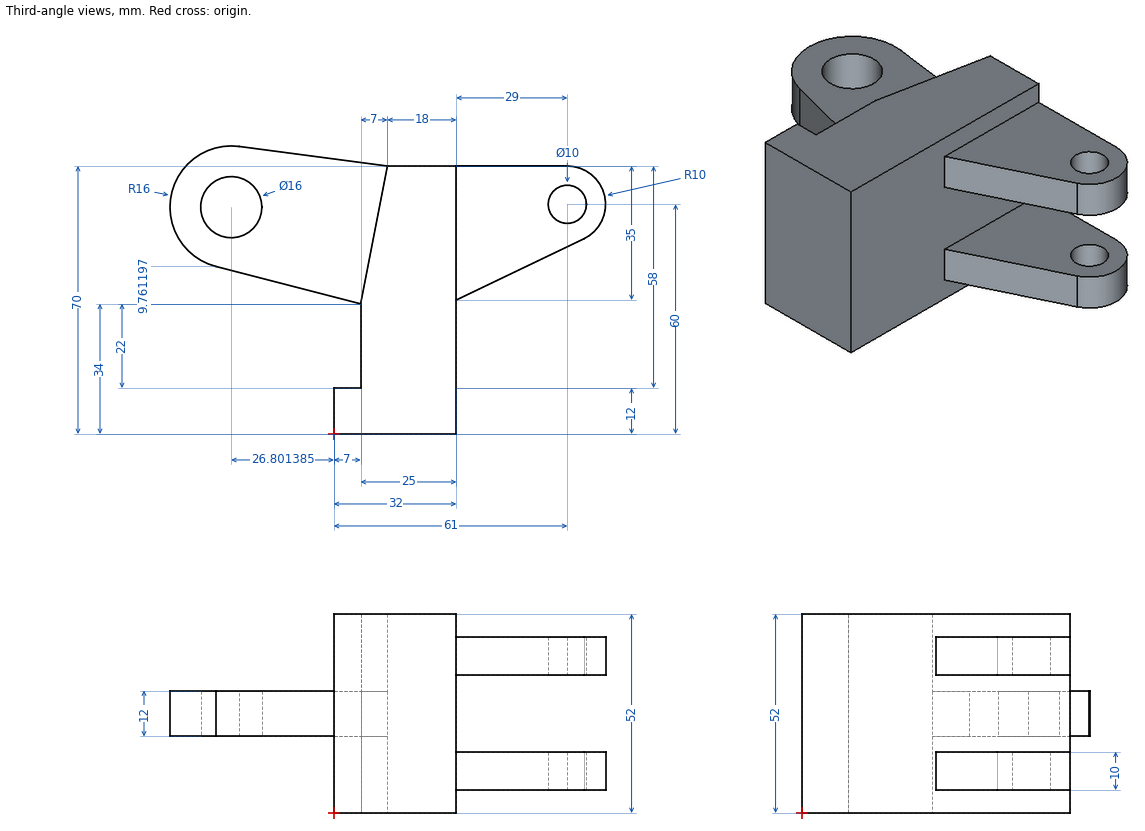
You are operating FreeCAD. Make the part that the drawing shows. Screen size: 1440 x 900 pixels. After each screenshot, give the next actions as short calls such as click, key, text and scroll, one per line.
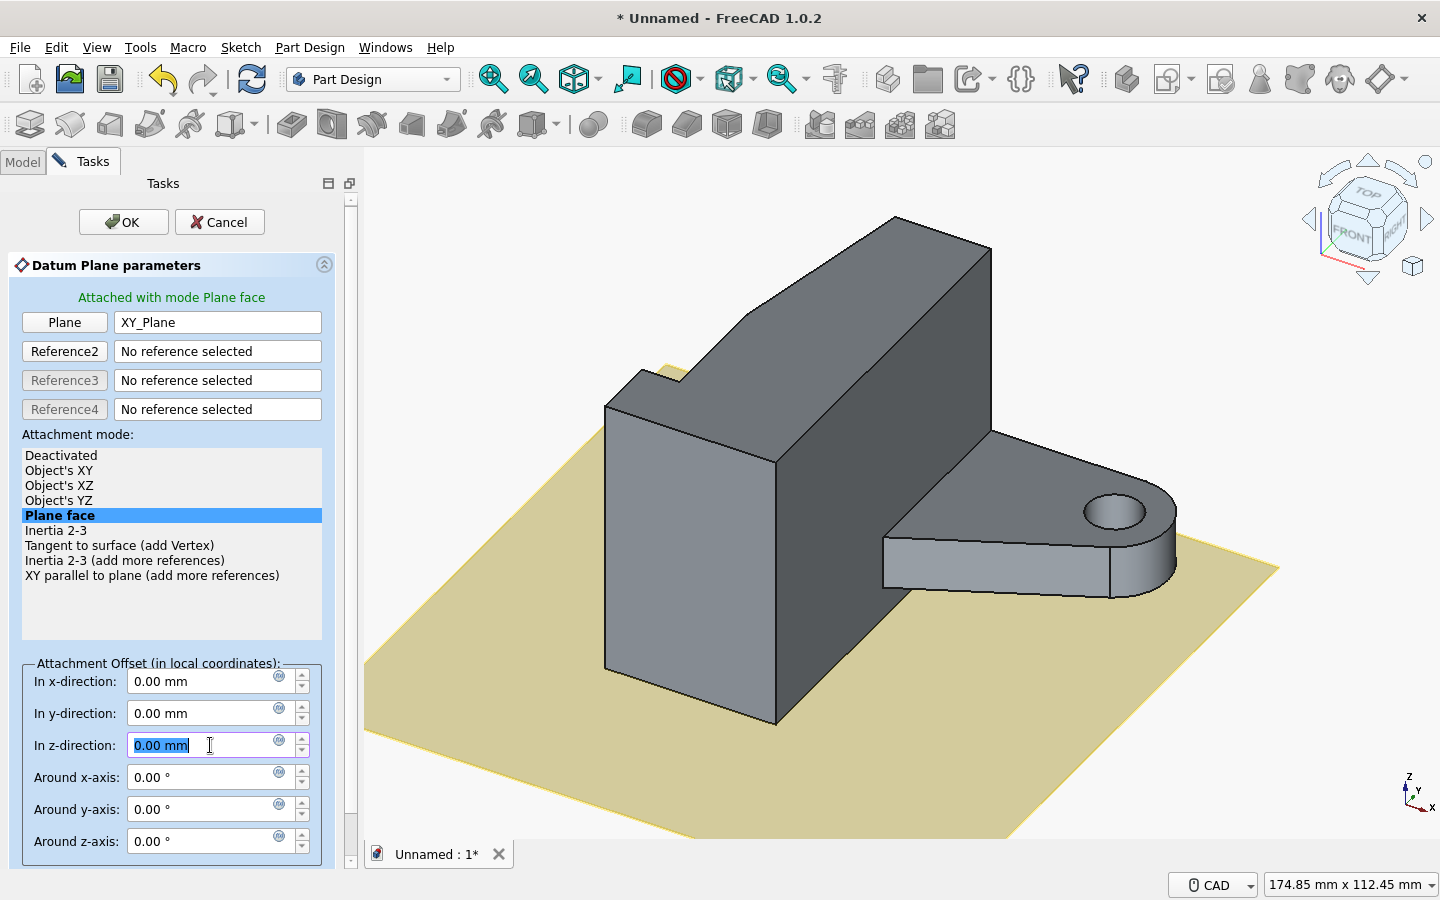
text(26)
key(Tab)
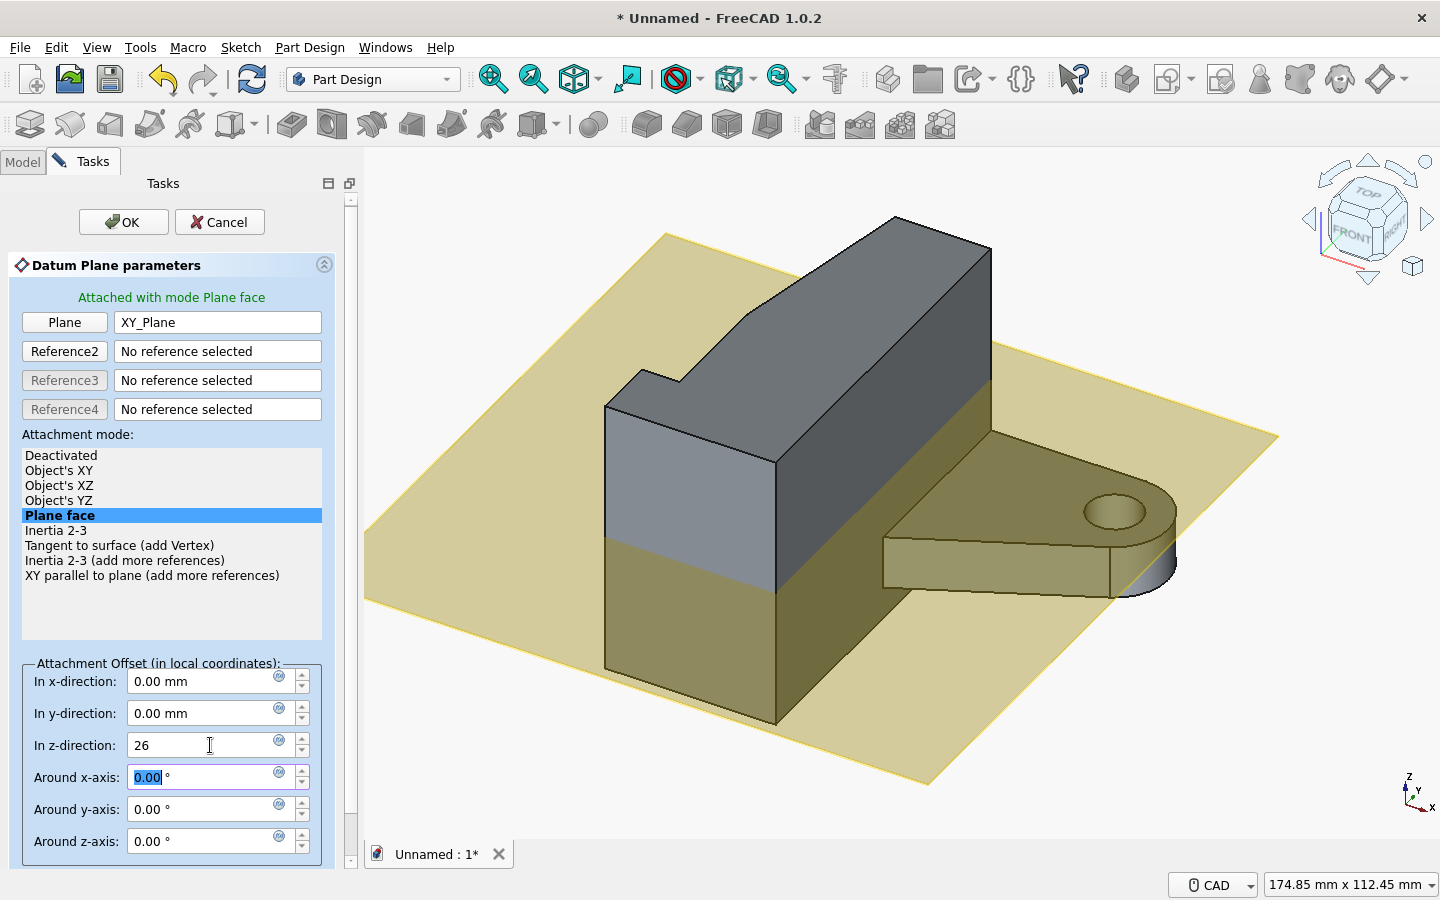
click(124, 222)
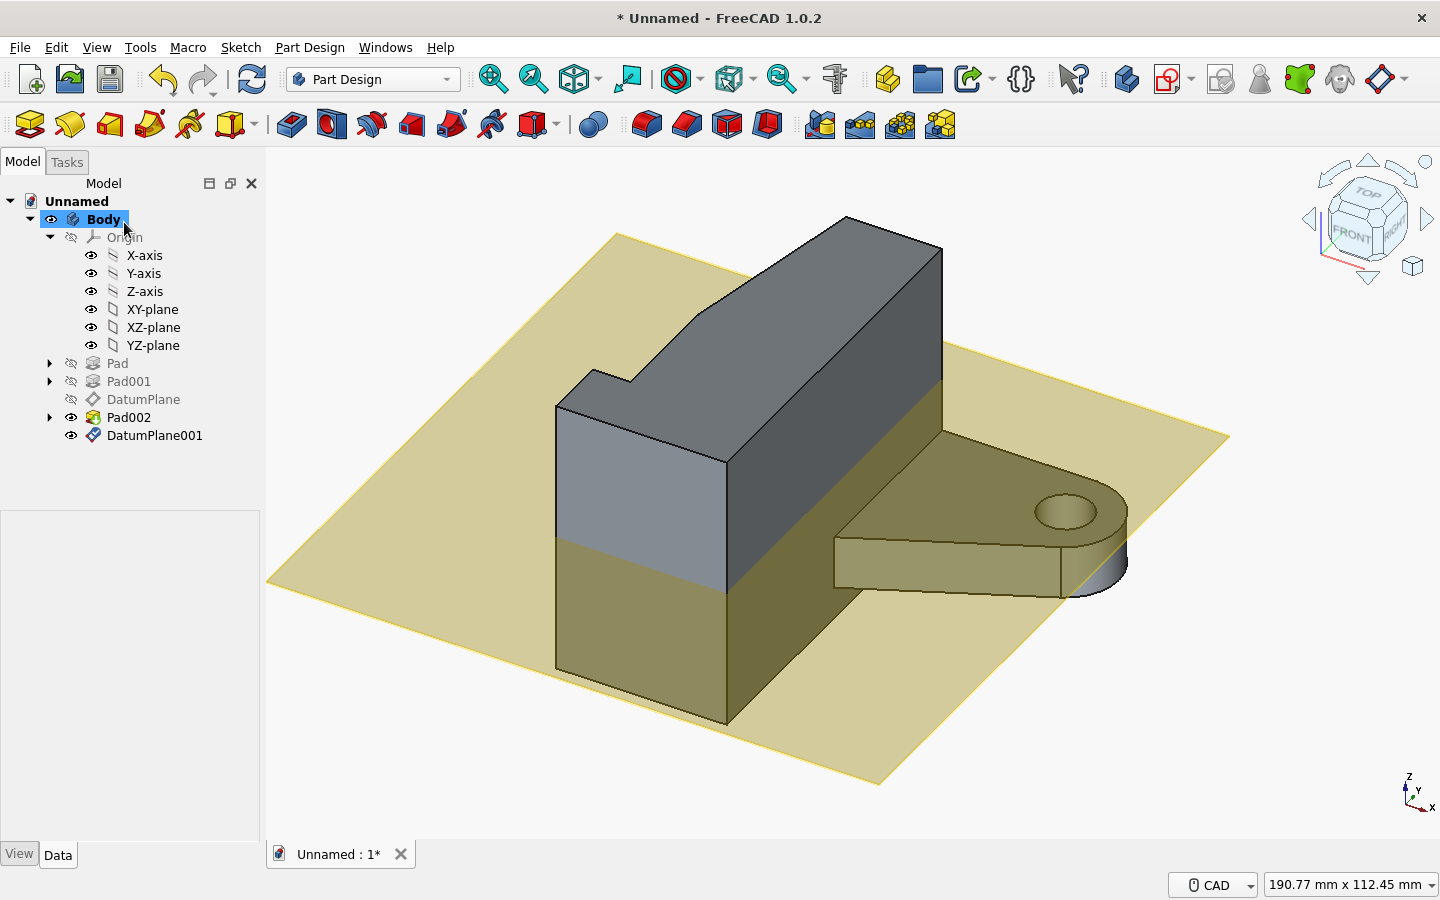
click(116, 417)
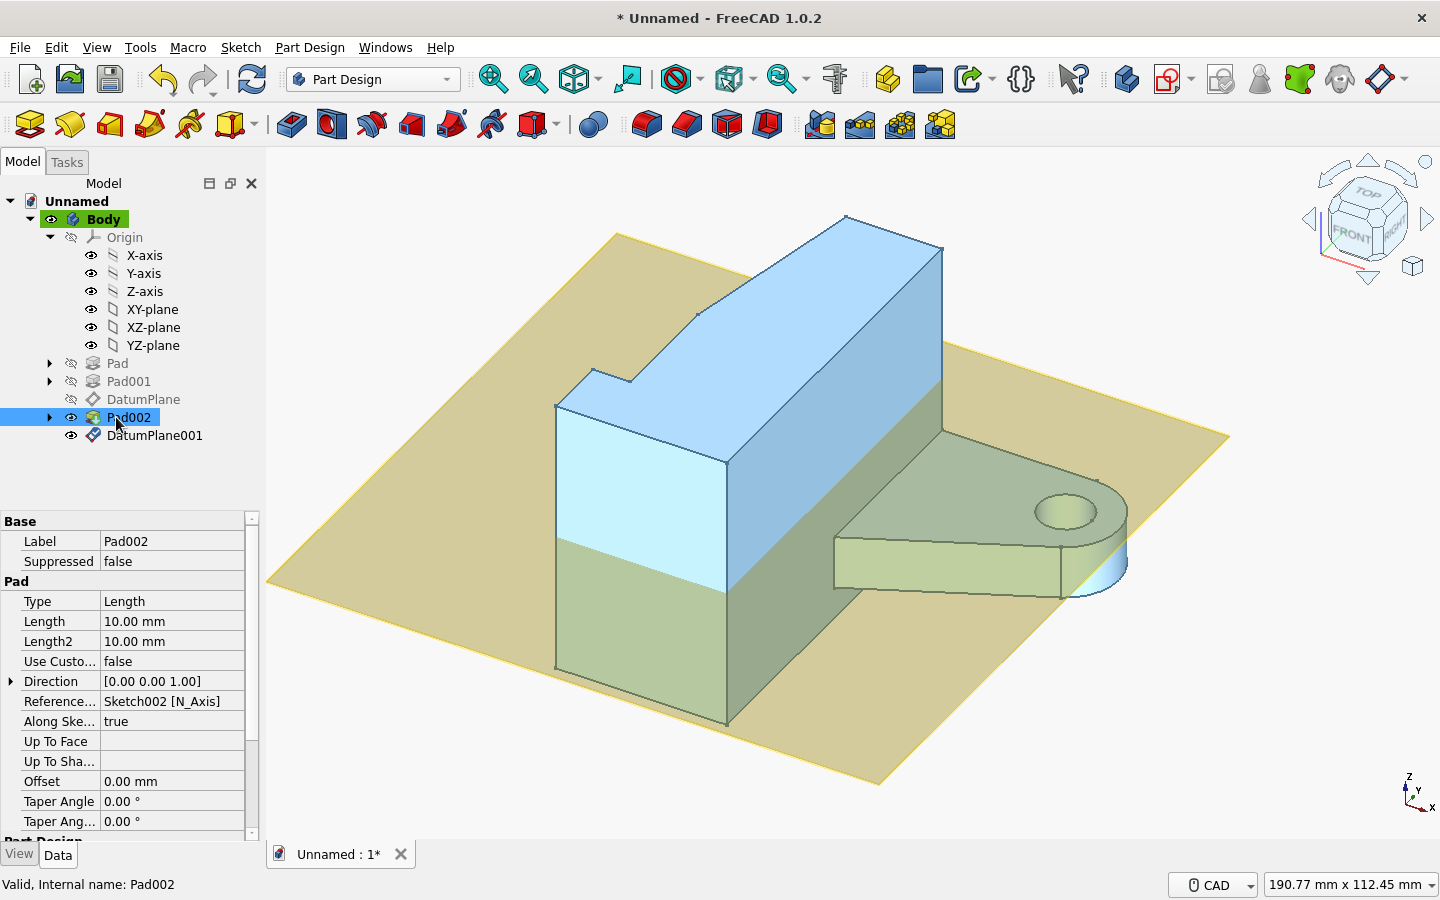
click(820, 124)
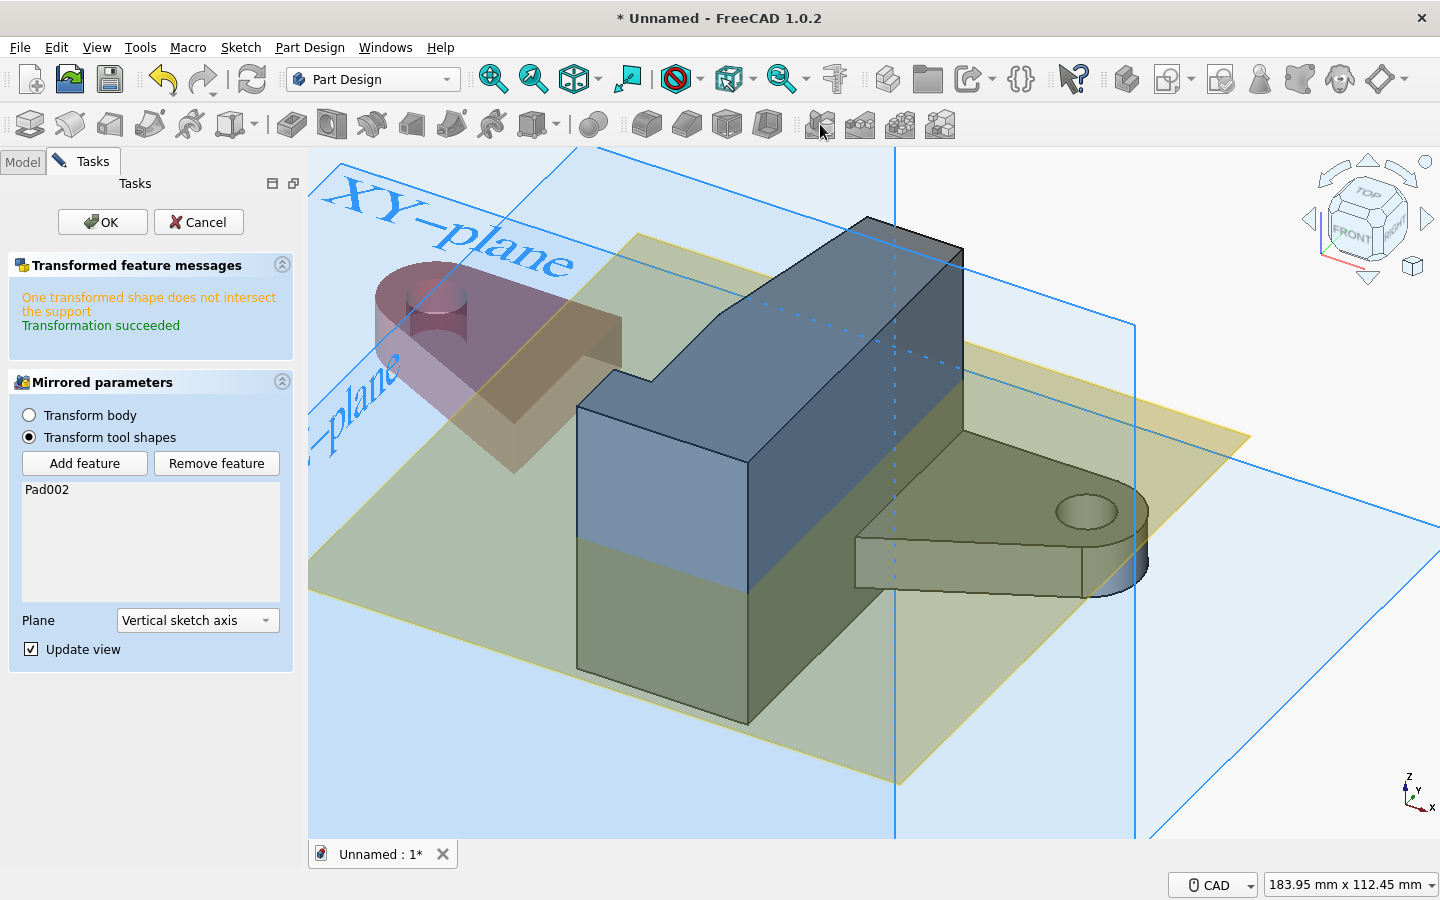
click(198, 620)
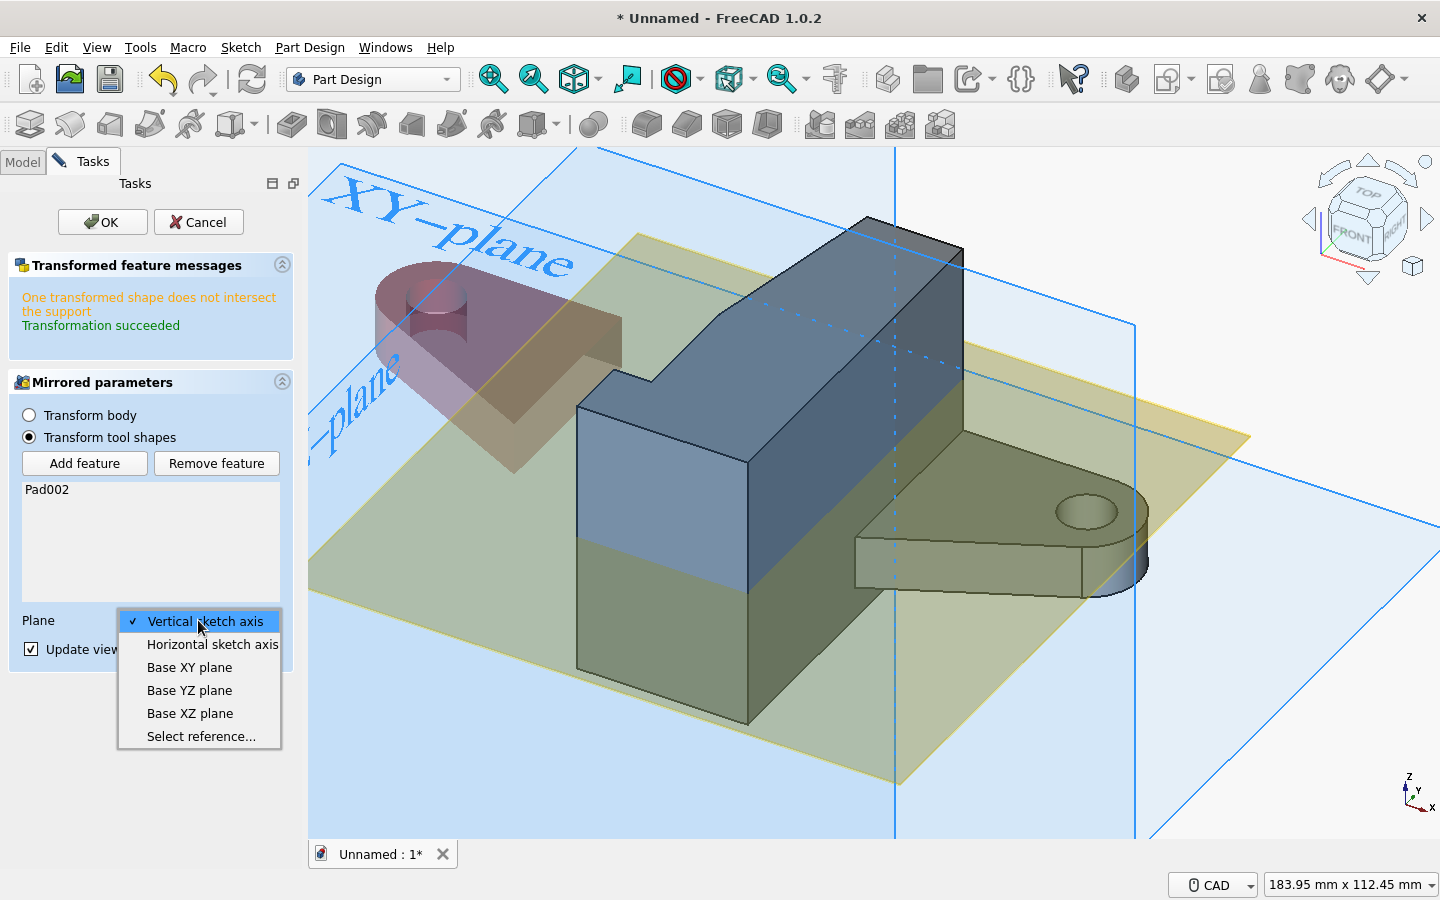
click(198, 736)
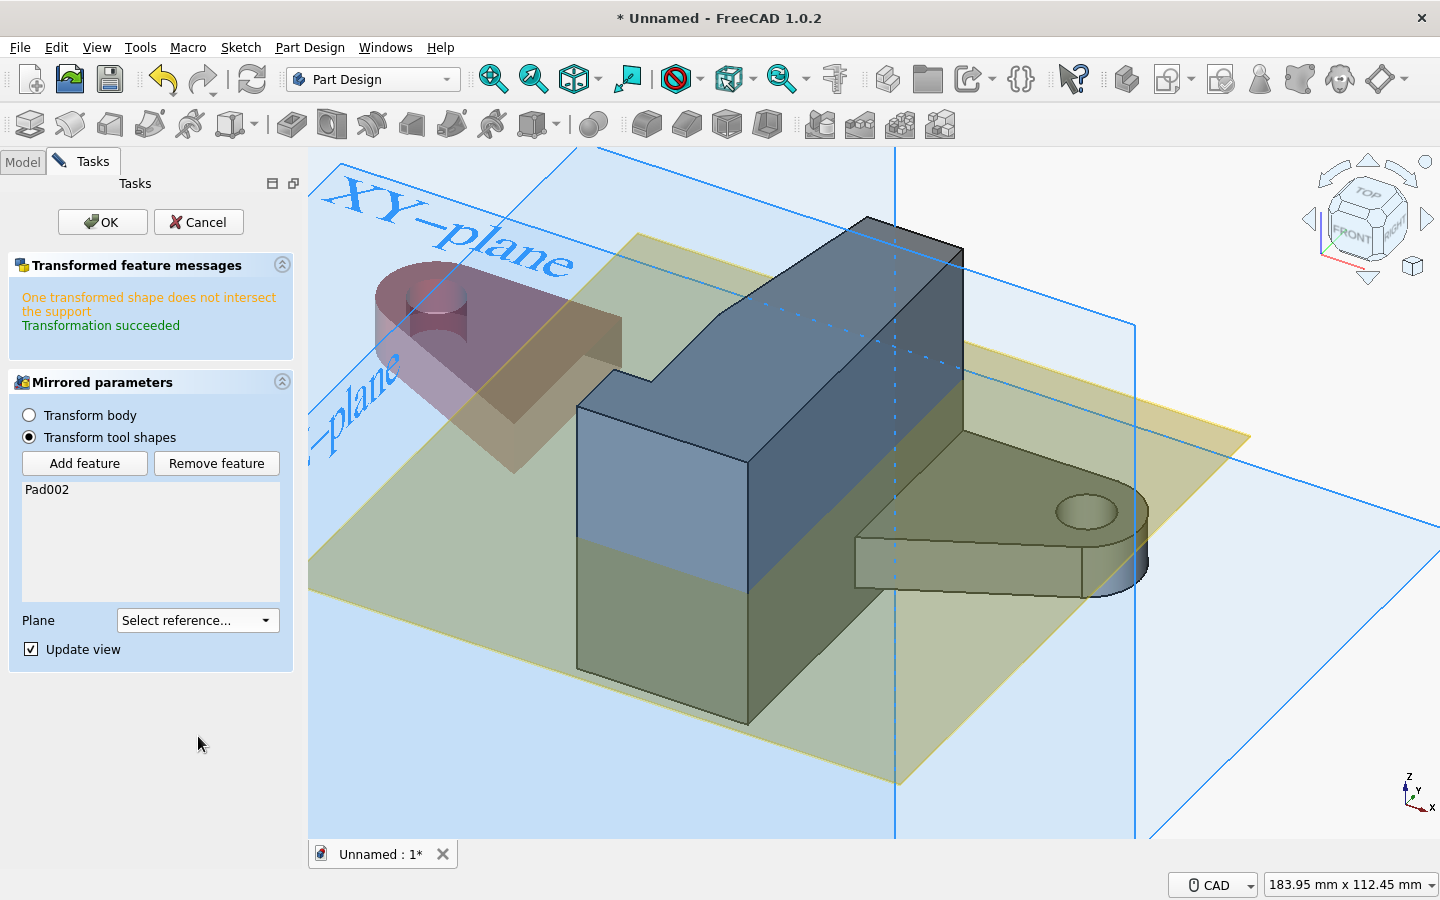
click(23, 161)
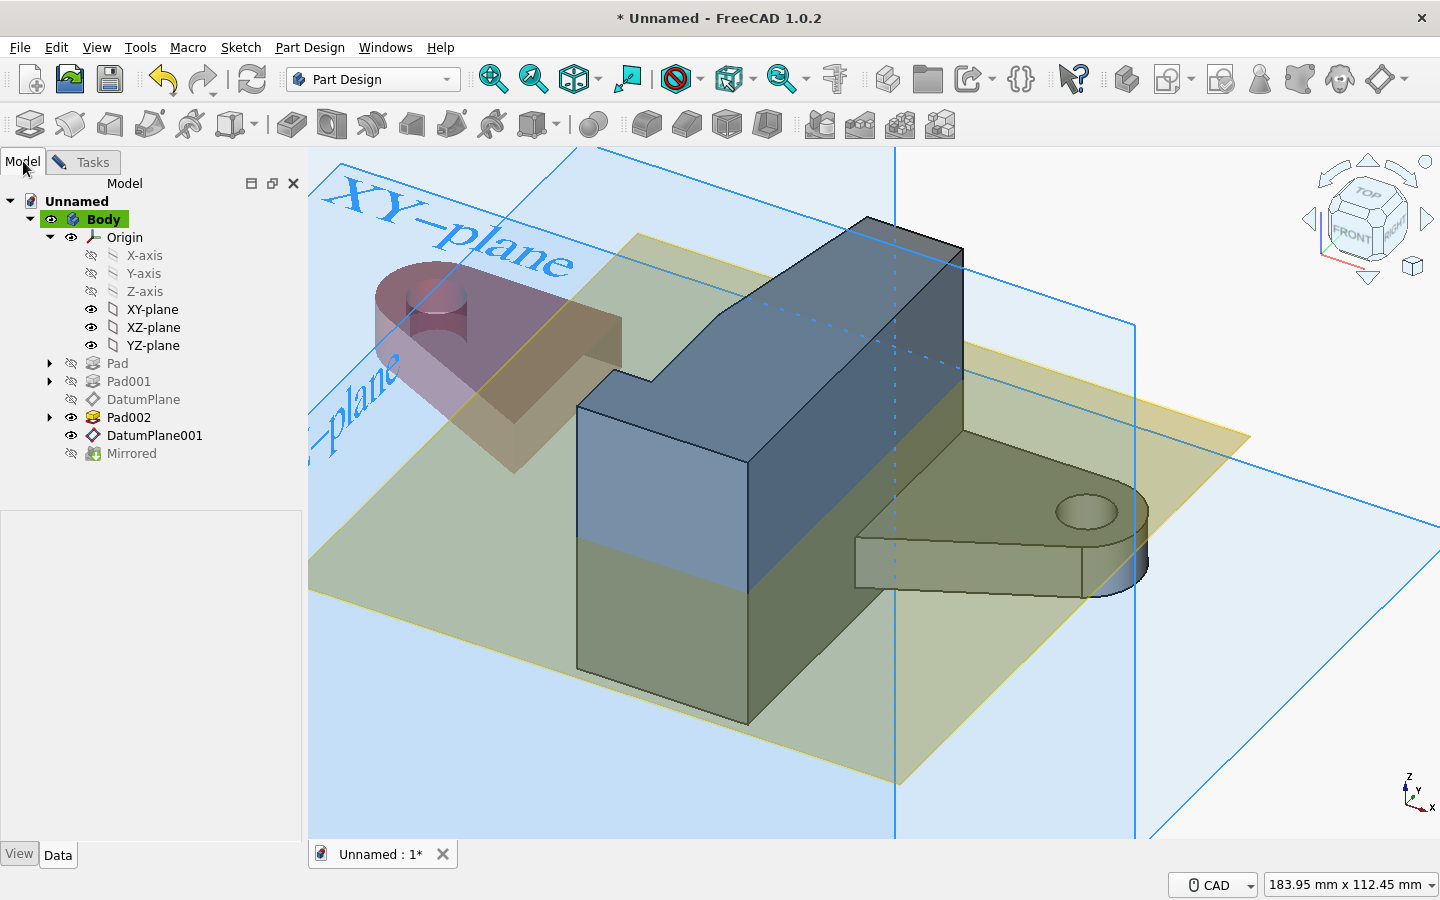
click(116, 435)